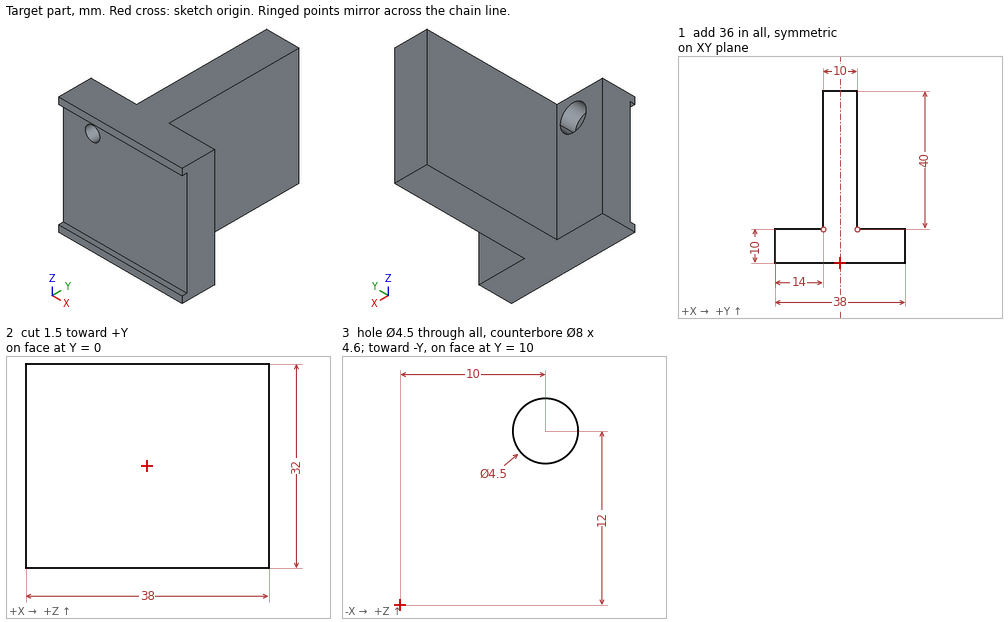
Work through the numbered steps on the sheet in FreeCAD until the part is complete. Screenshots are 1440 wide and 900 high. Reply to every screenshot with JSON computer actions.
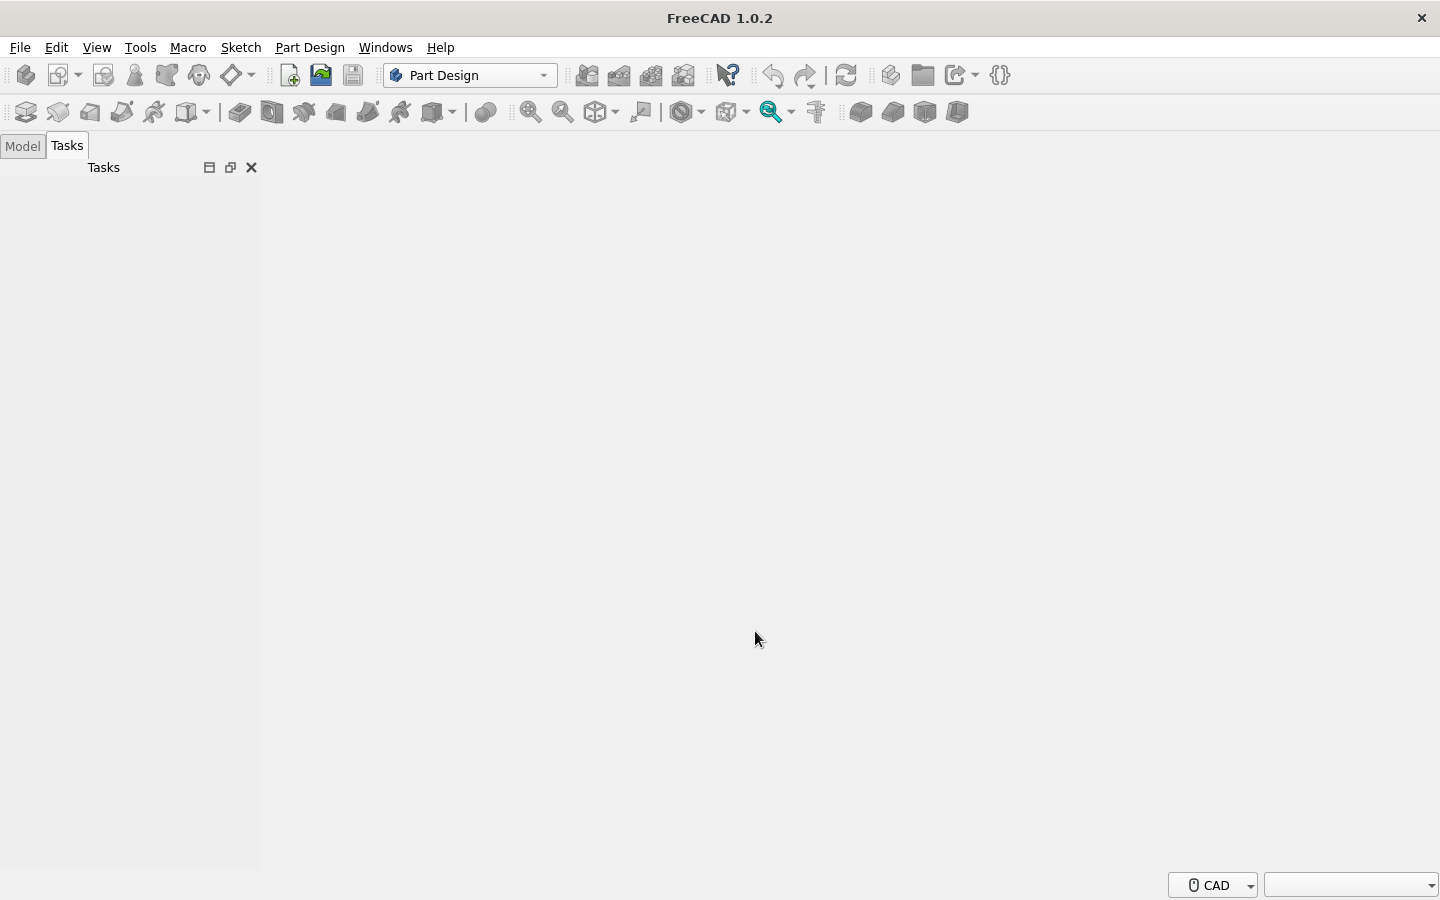
{"action": "left_click", "coordinate": [290, 76]}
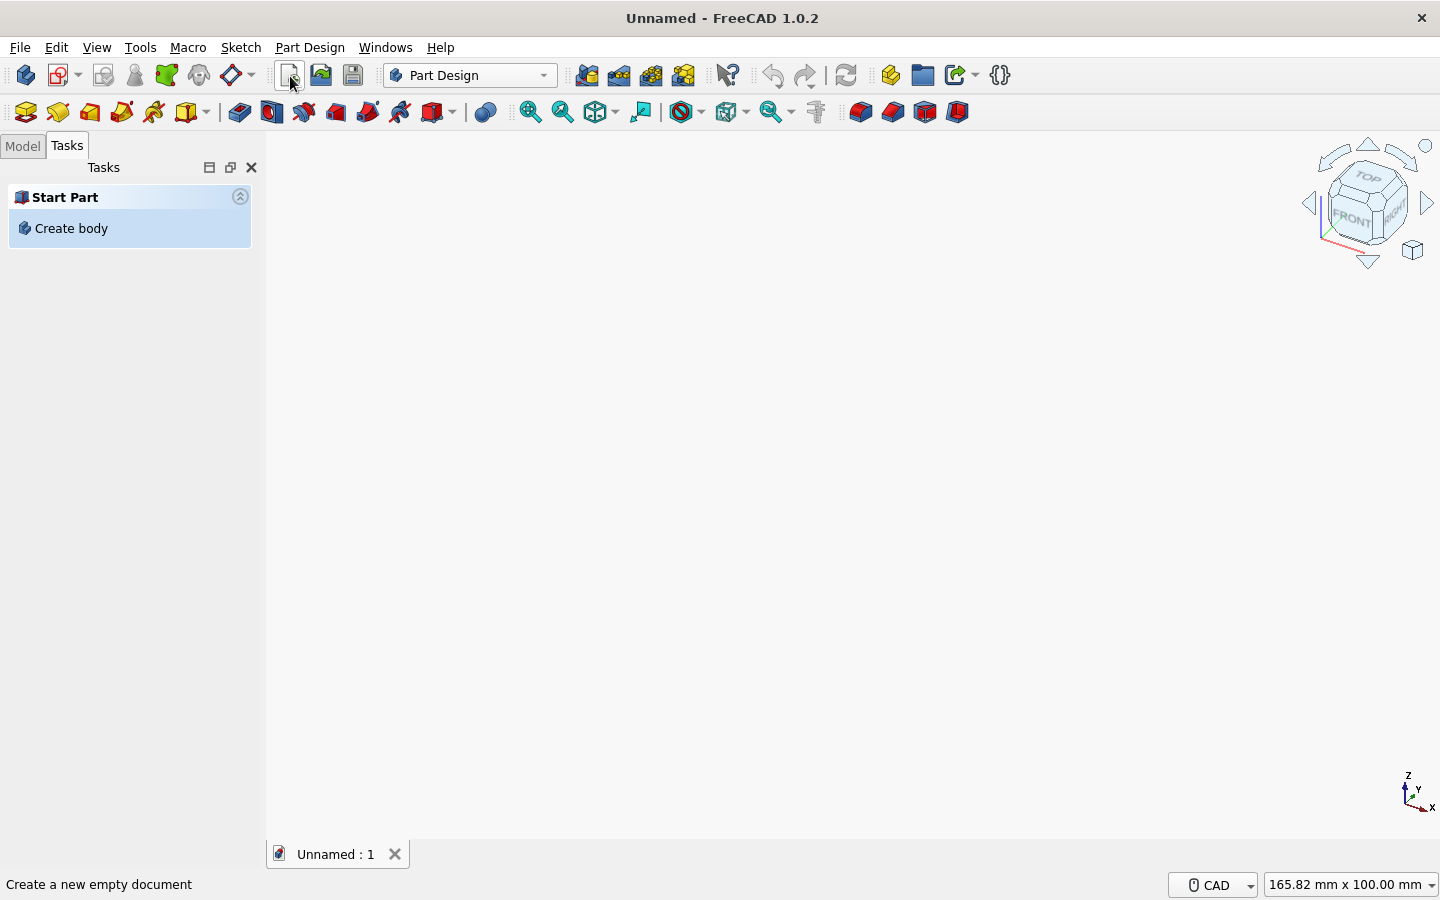
{"action": "left_click", "coordinate": [58, 76]}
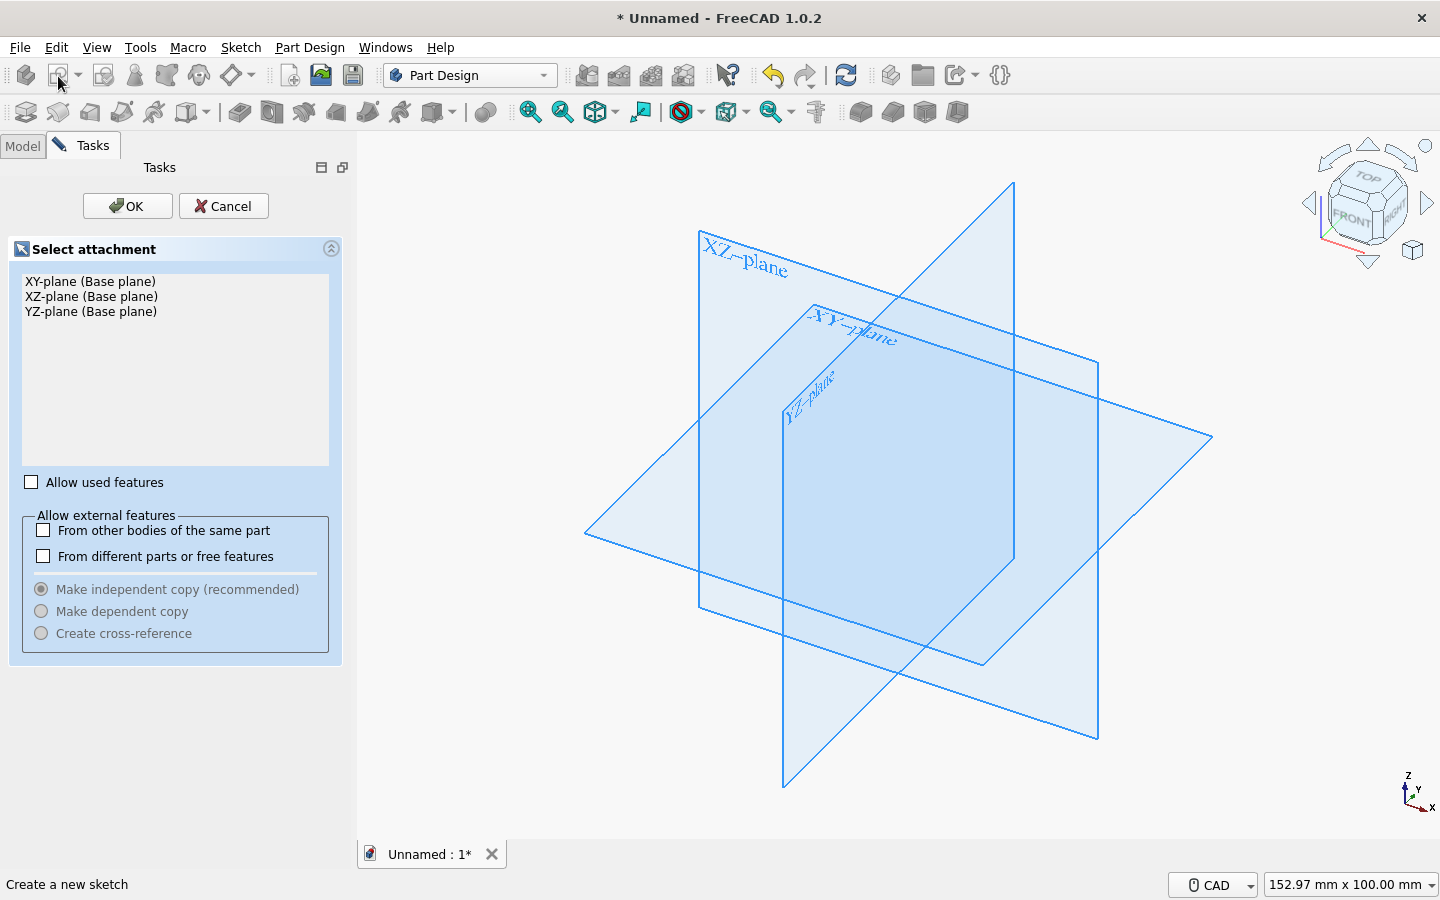
{"action": "left_click", "coordinate": [82, 282]}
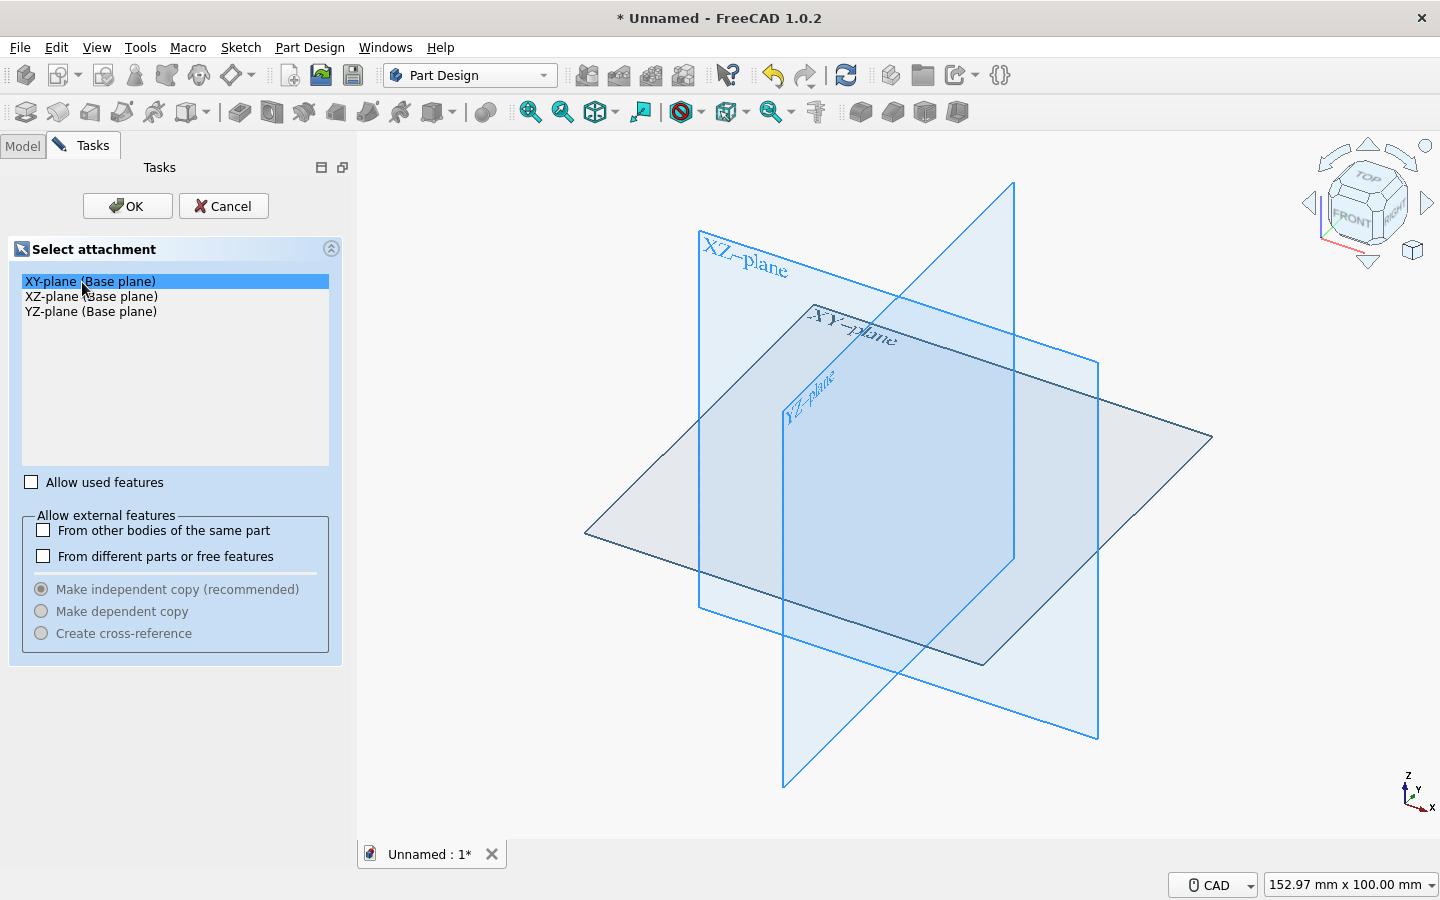
{"action": "left_click", "coordinate": [128, 206]}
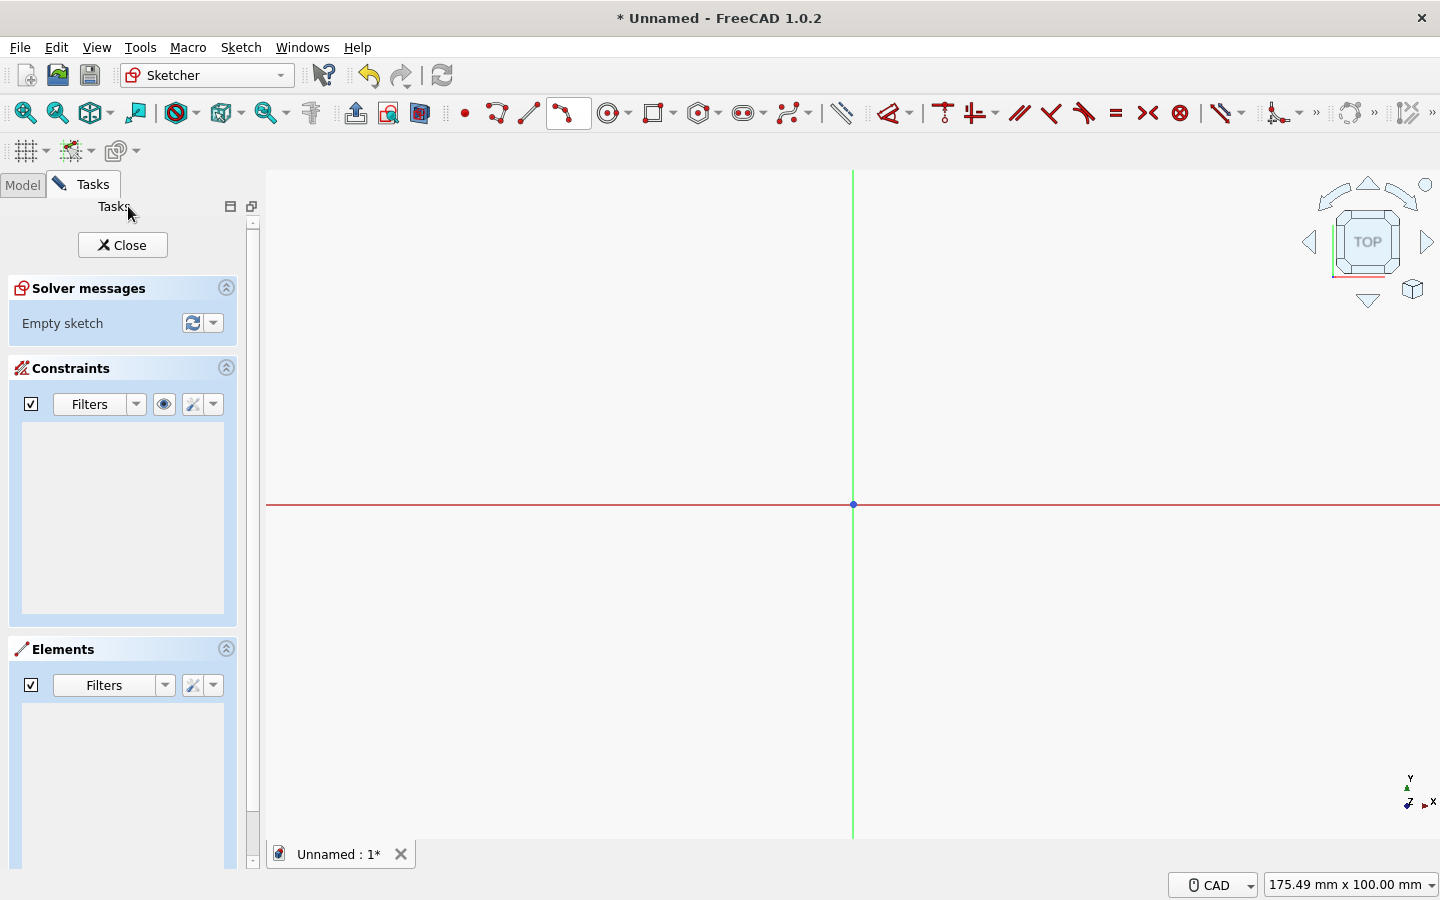
{"action": "scroll", "coordinate": [475, 811], "scroll_direction": "down", "scroll_amount": 1}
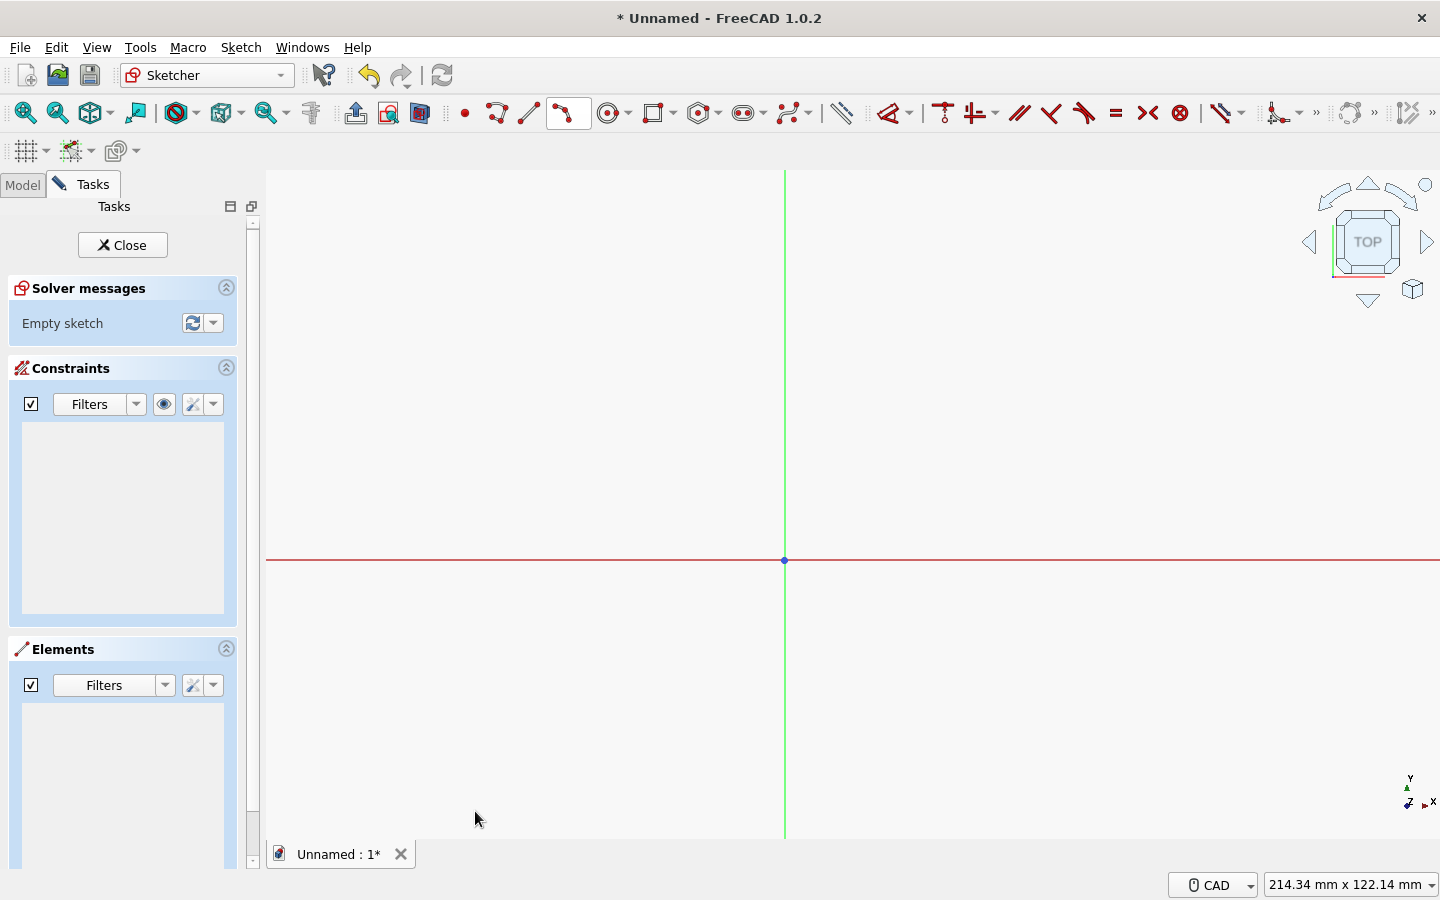
{"action": "scroll", "coordinate": [785, 258], "scroll_direction": "up", "scroll_amount": 2}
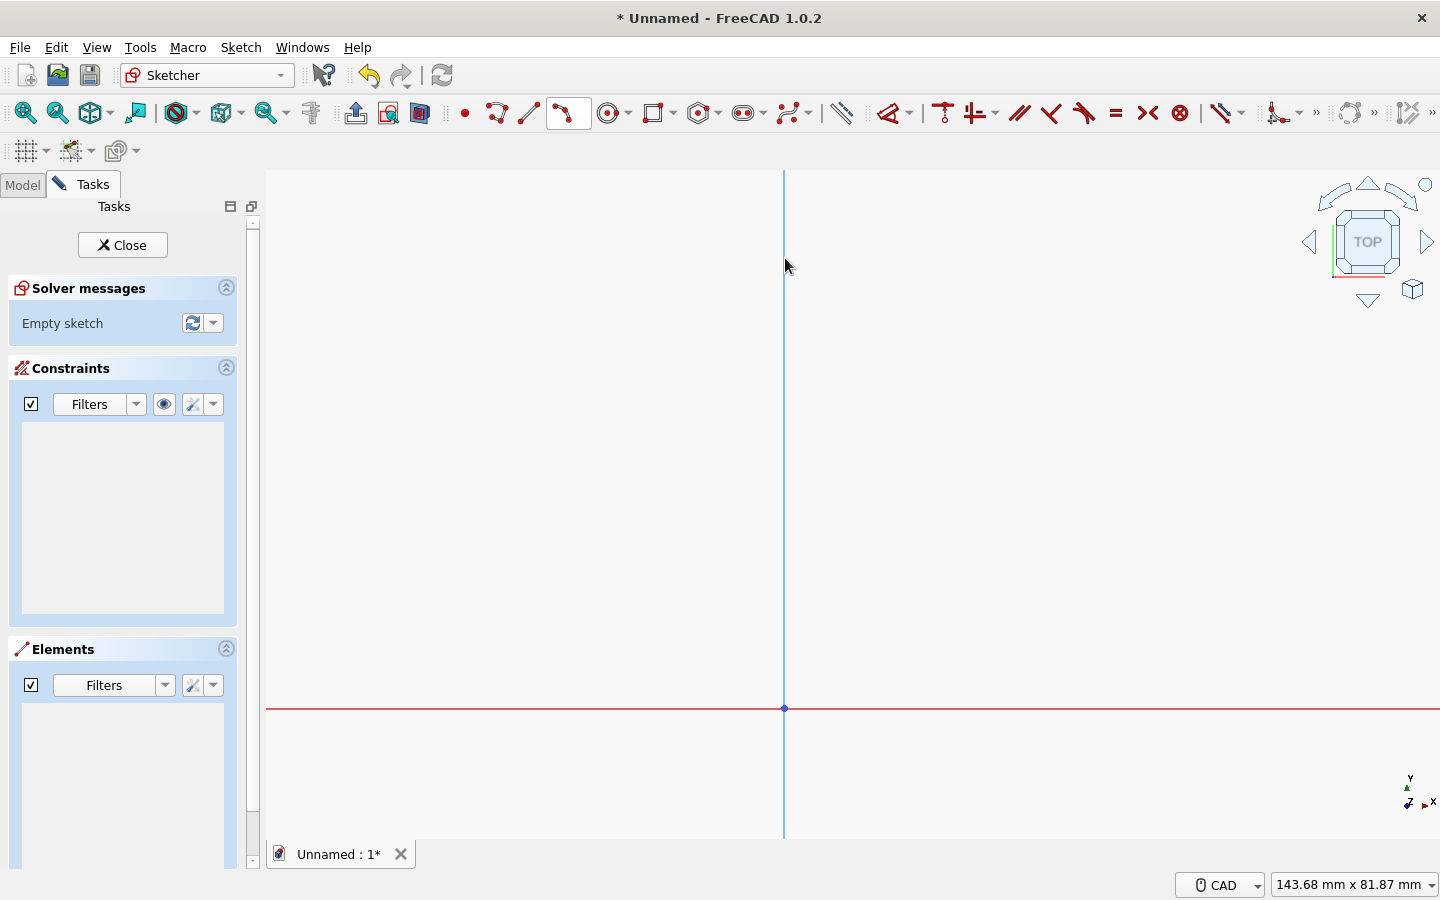
{"action": "left_click", "coordinate": [498, 114]}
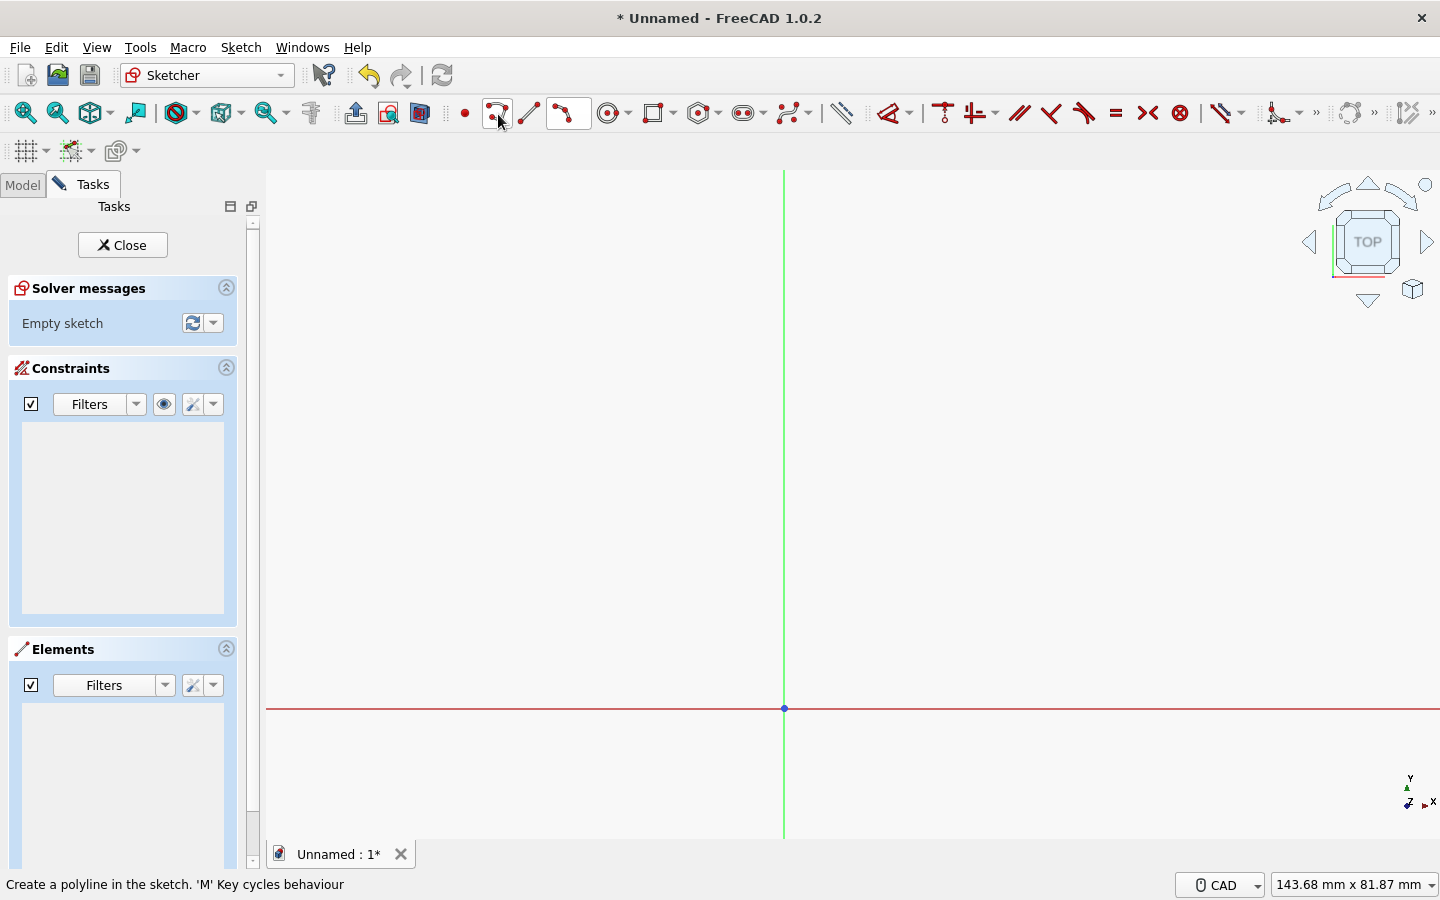
{"action": "left_click", "coordinate": [825, 627]}
{"action": "left_click", "coordinate": [825, 300]}
{"action": "left_click", "coordinate": [743, 300]}
{"action": "left_click", "coordinate": [743, 627]}
{"action": "left_click", "coordinate": [629, 627]}
{"action": "left_click", "coordinate": [629, 709]}
{"action": "left_click", "coordinate": [939, 700]}
{"action": "left_click", "coordinate": [939, 627]}
{"action": "left_click", "coordinate": [825, 628]}
{"action": "key", "text": "Escape"}
{"action": "key", "text": "Escape"}